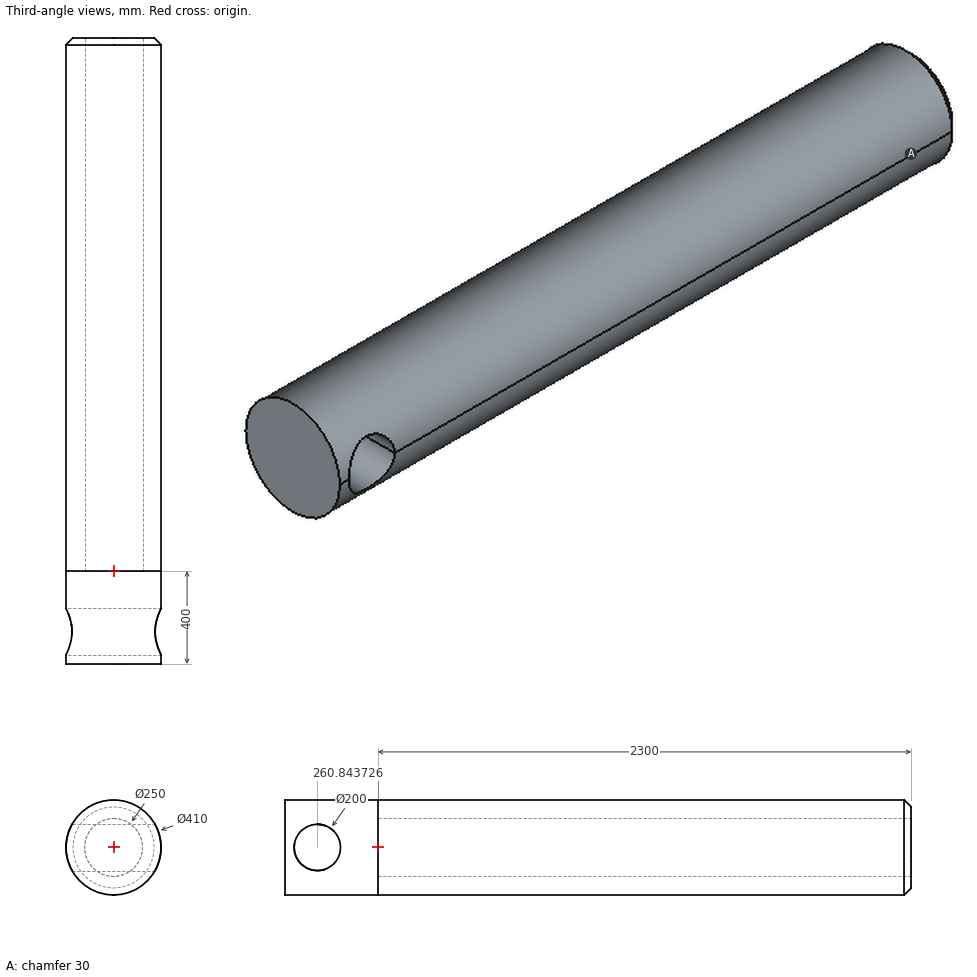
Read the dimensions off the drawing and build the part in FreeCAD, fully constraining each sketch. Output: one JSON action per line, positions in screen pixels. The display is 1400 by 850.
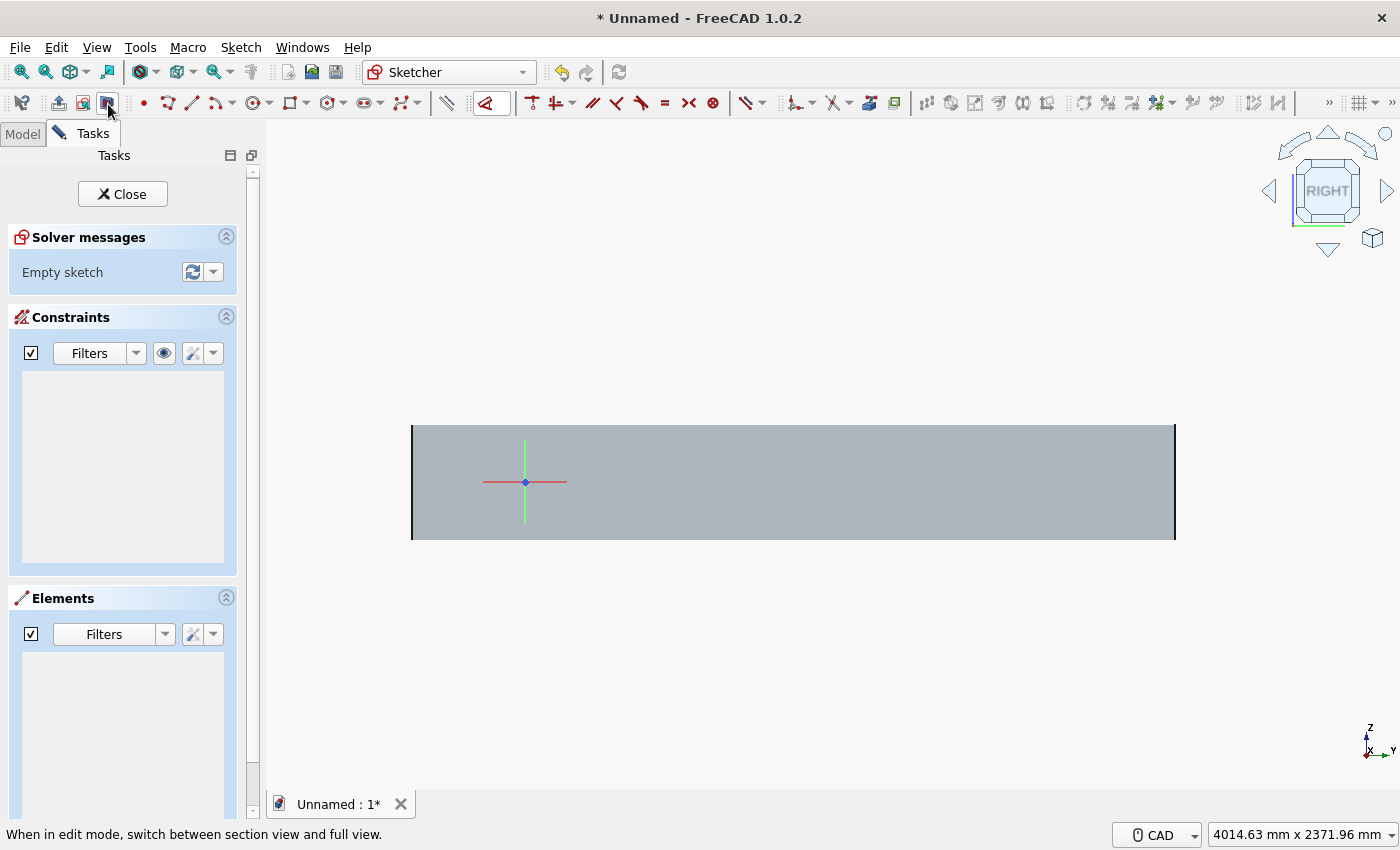
{"action": "scroll", "coordinate": [417, 488], "scroll_direction": "up", "scroll_amount": 9}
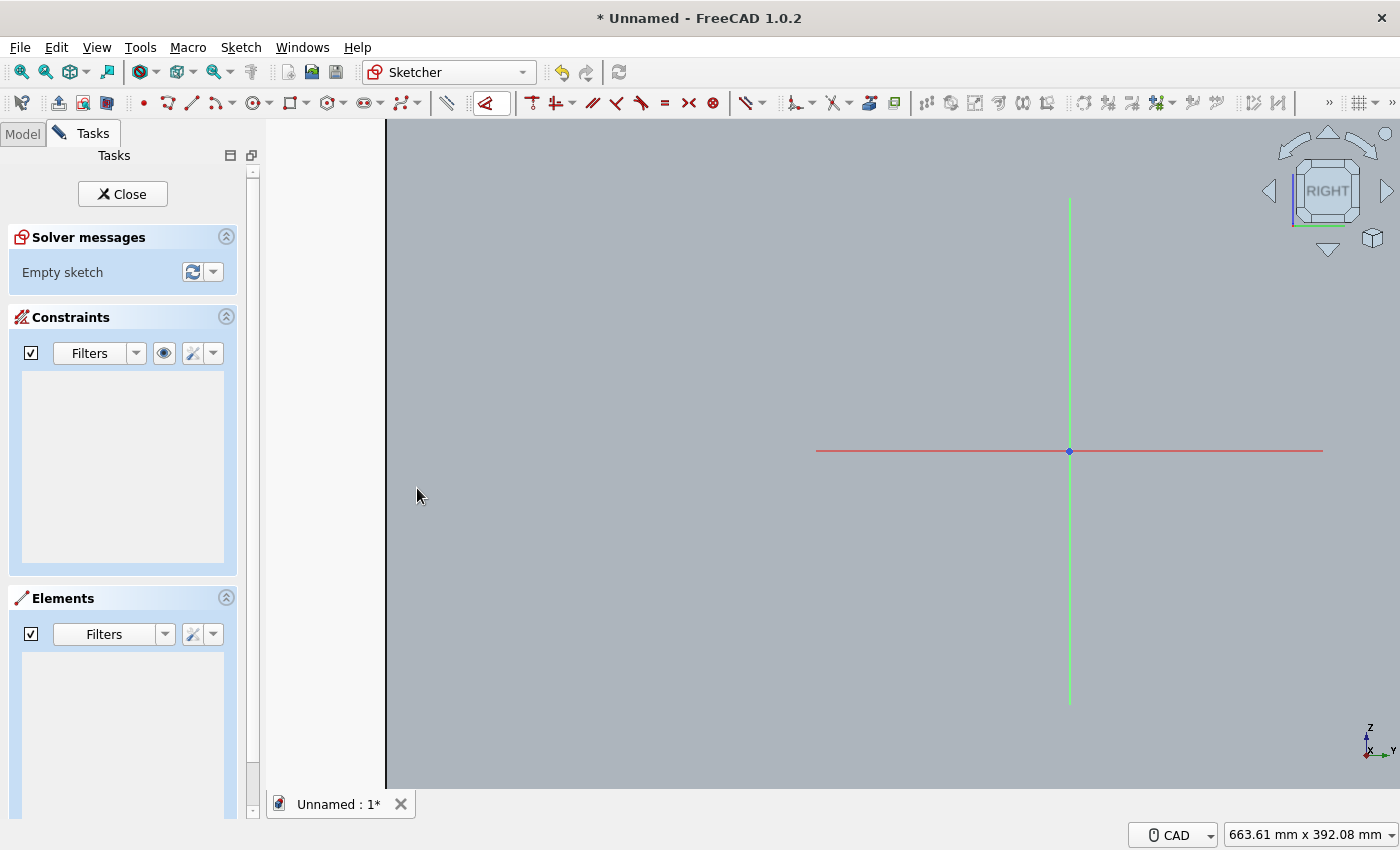
{"action": "left_click", "coordinate": [254, 104]}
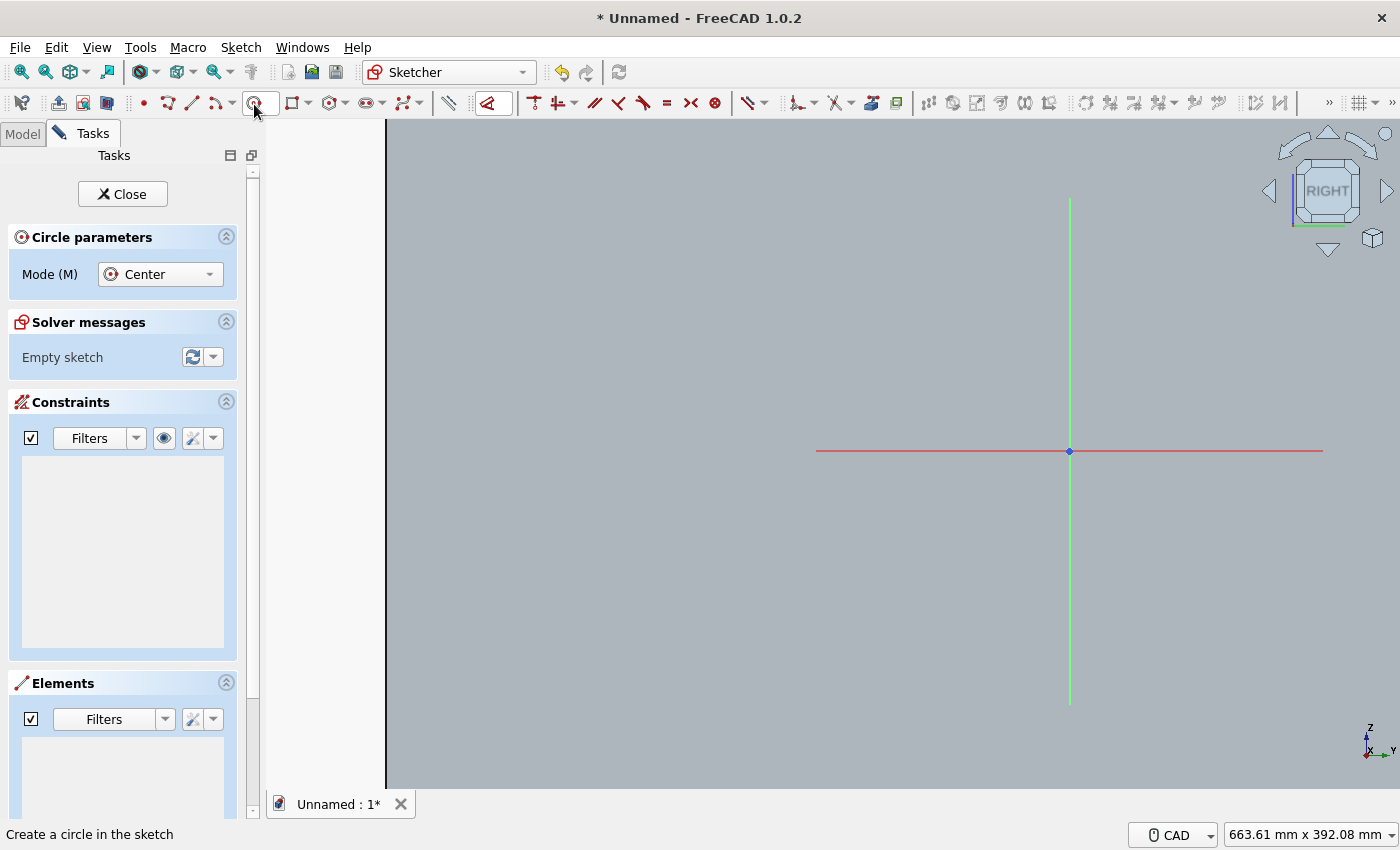
{"action": "left_click", "coordinate": [624, 451]}
{"action": "mouse_move", "coordinate": [745, 330]}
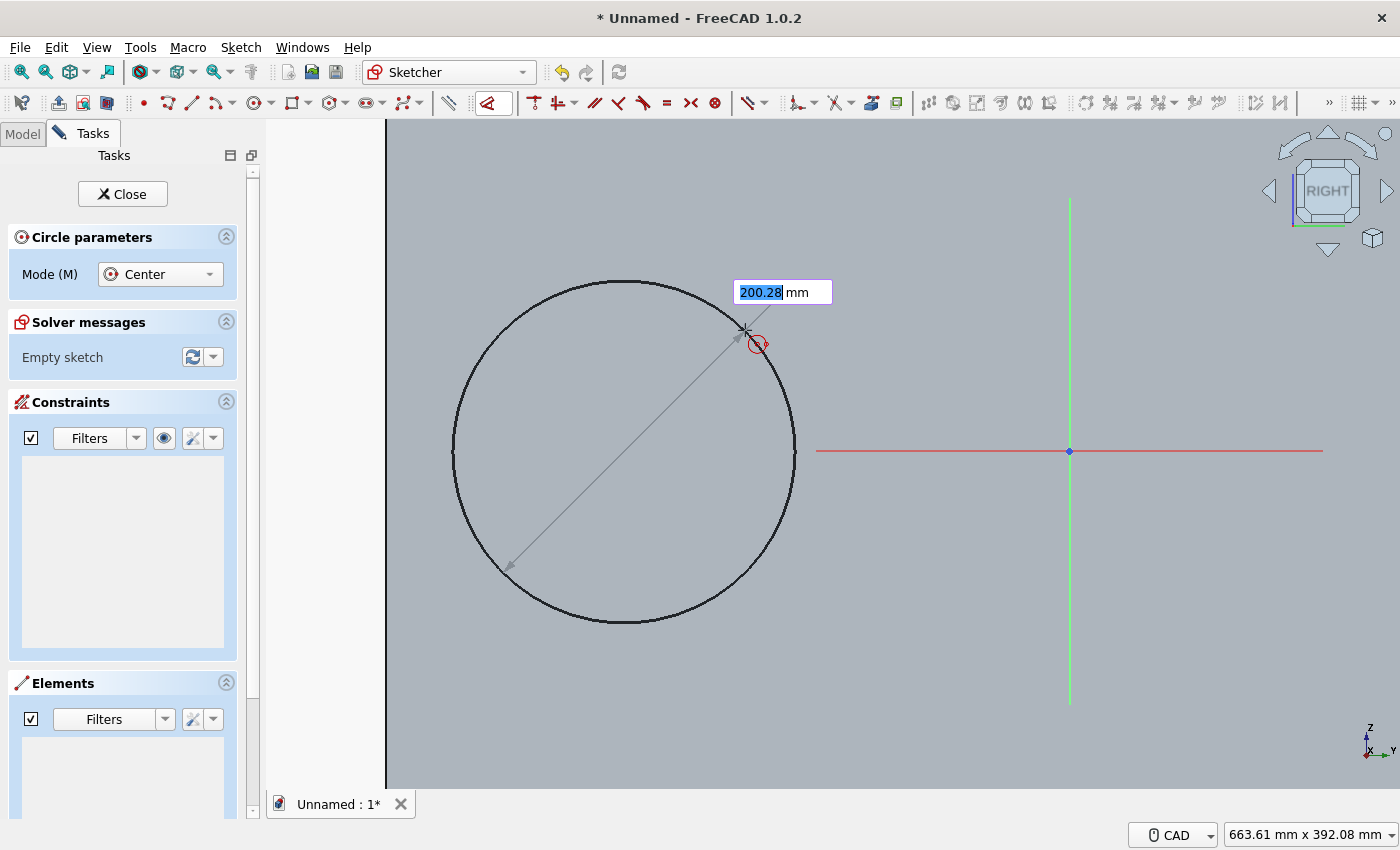
{"action": "type", "text": "200"}
{"action": "key", "text": "Return"}
{"action": "key", "text": "Escape"}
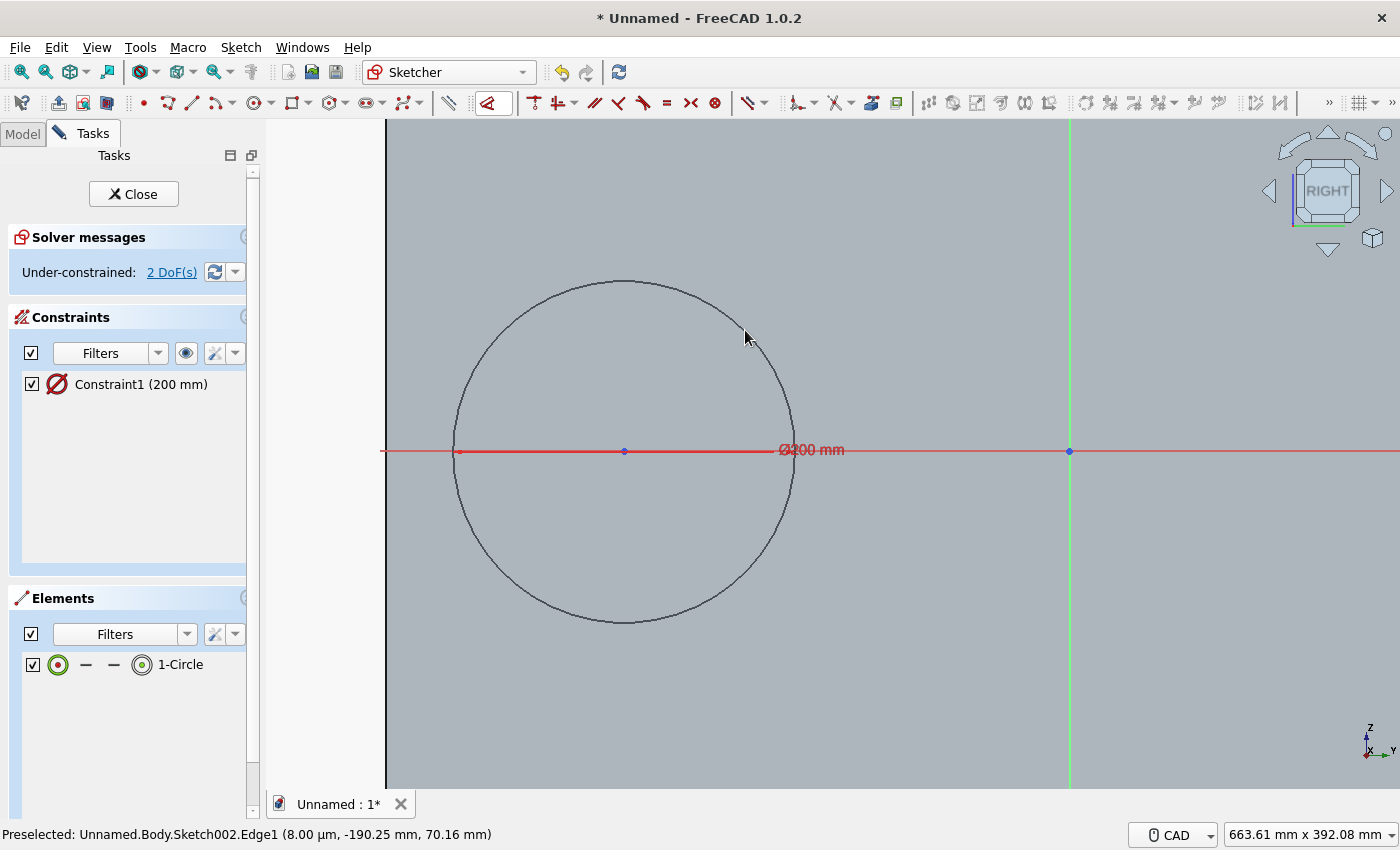
{"action": "left_click", "coordinate": [624, 452]}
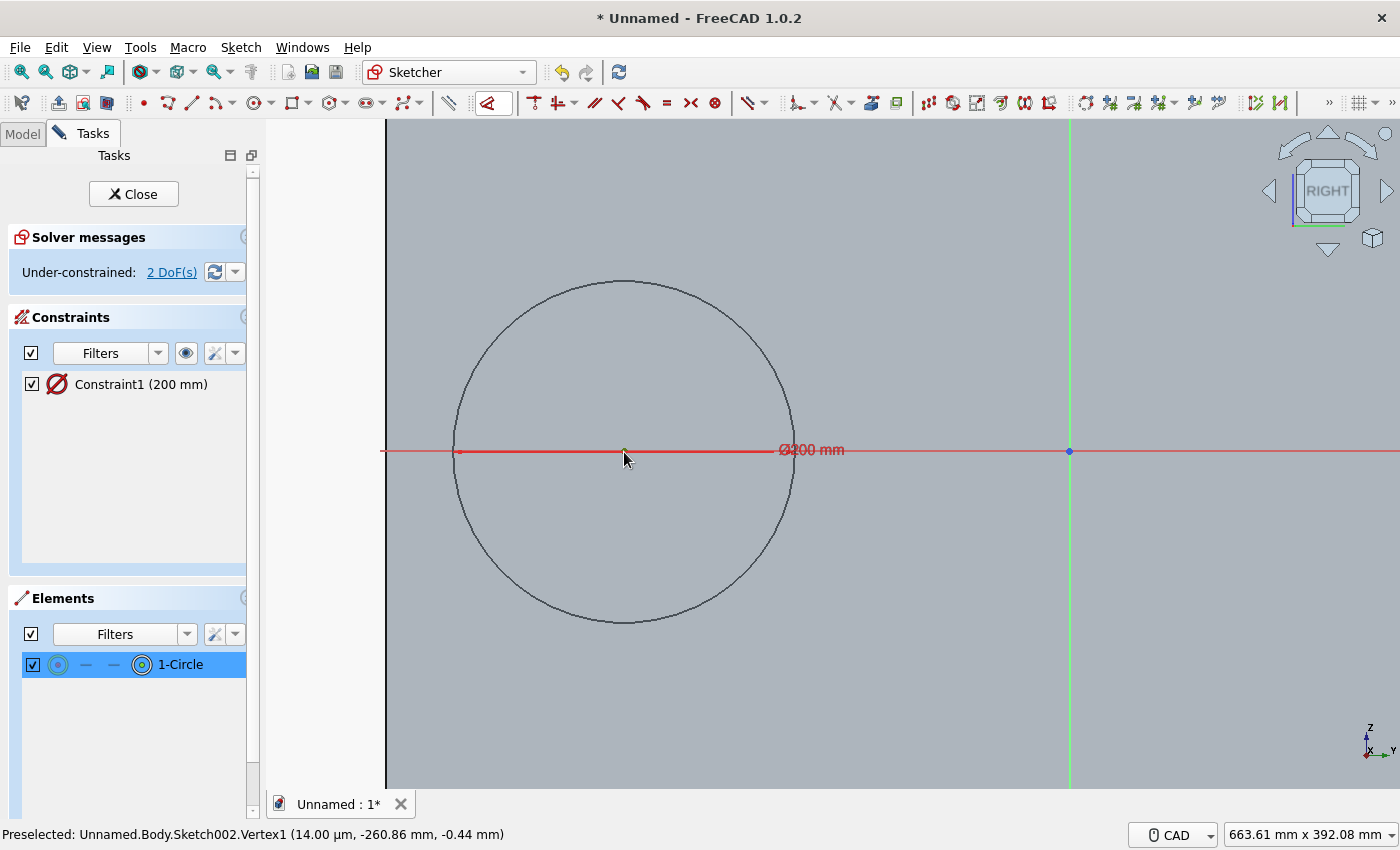
{"action": "left_click", "coordinate": [496, 451]}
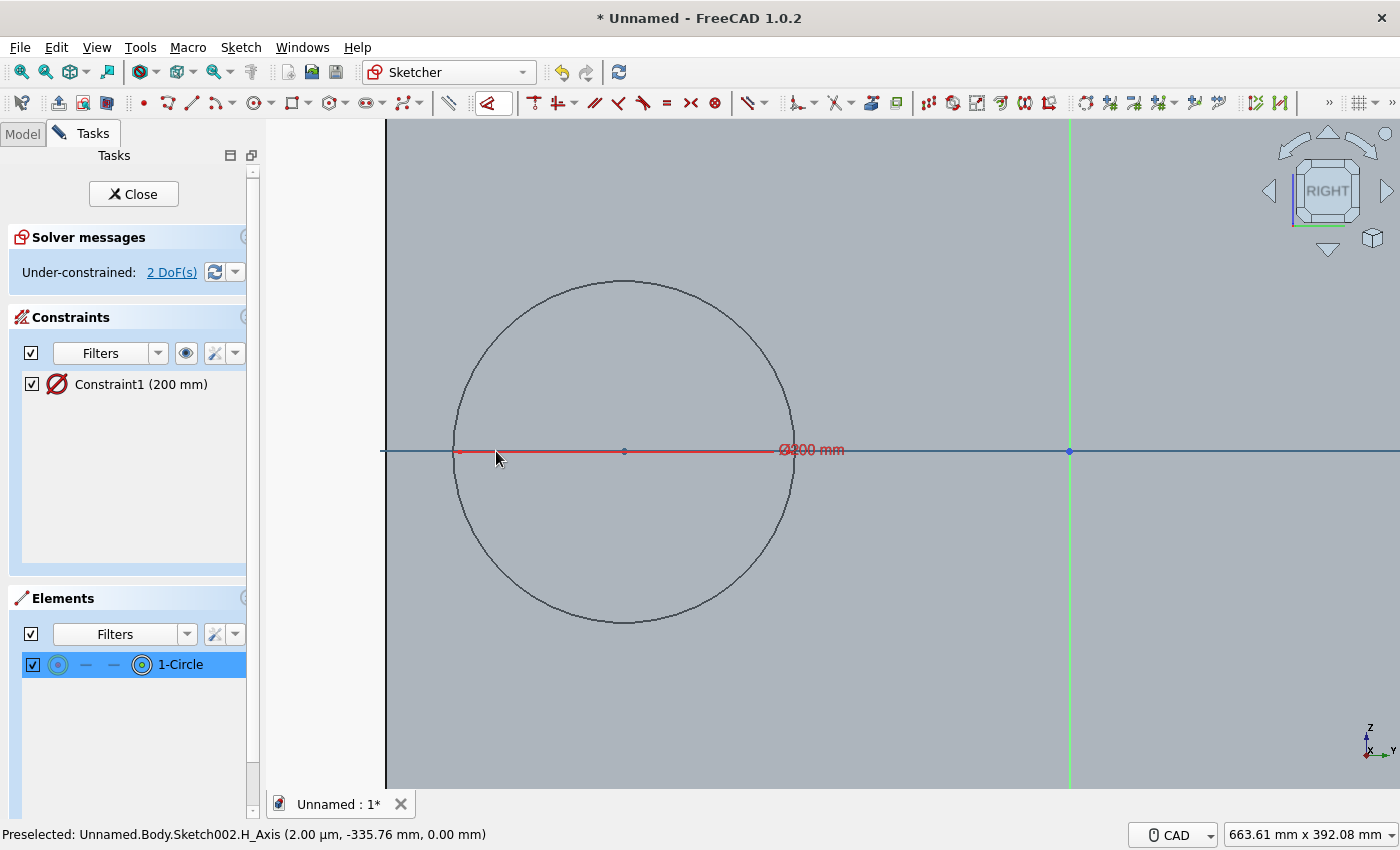
{"action": "left_click", "coordinate": [534, 104]}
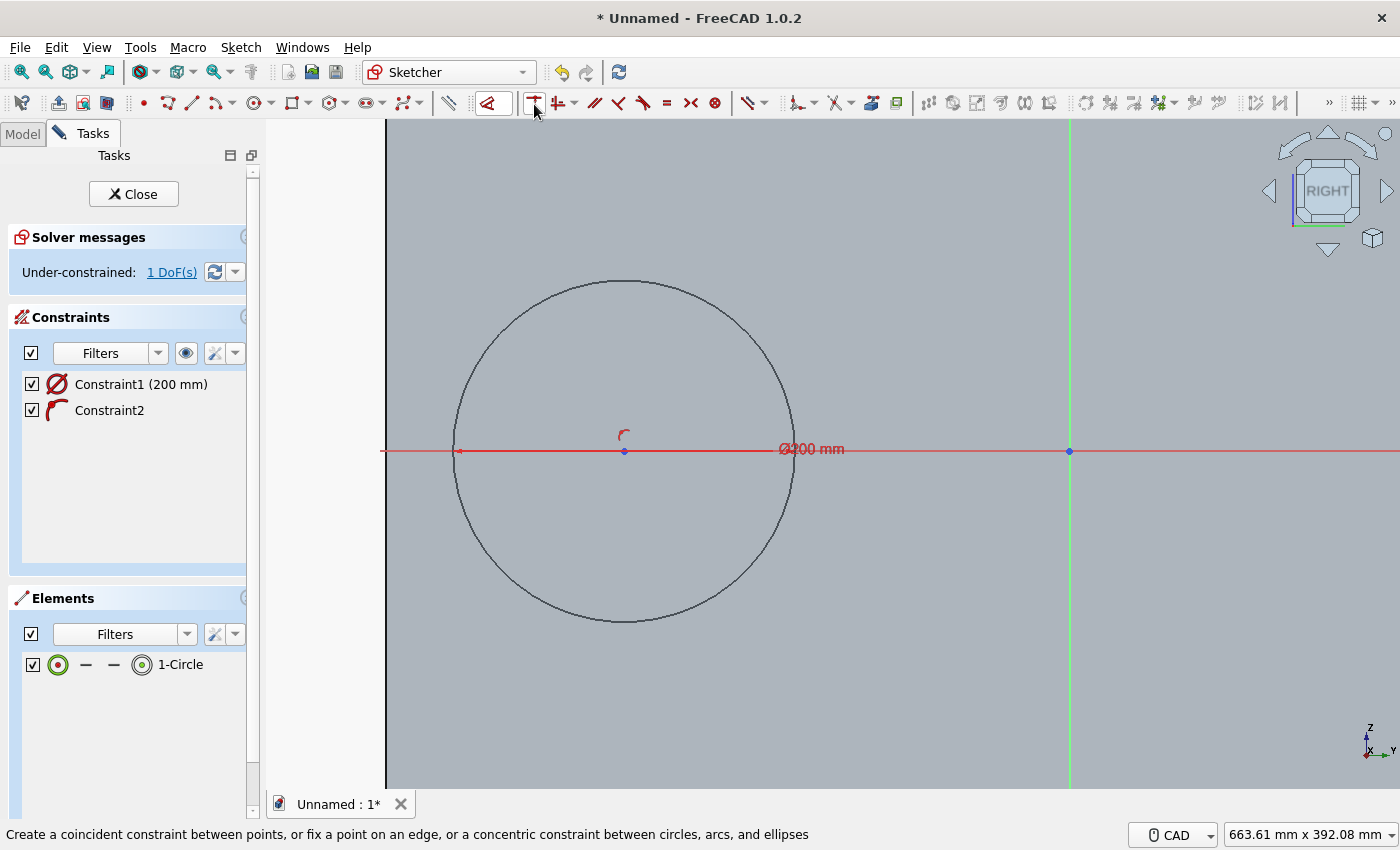
{"action": "left_click", "coordinate": [488, 104]}